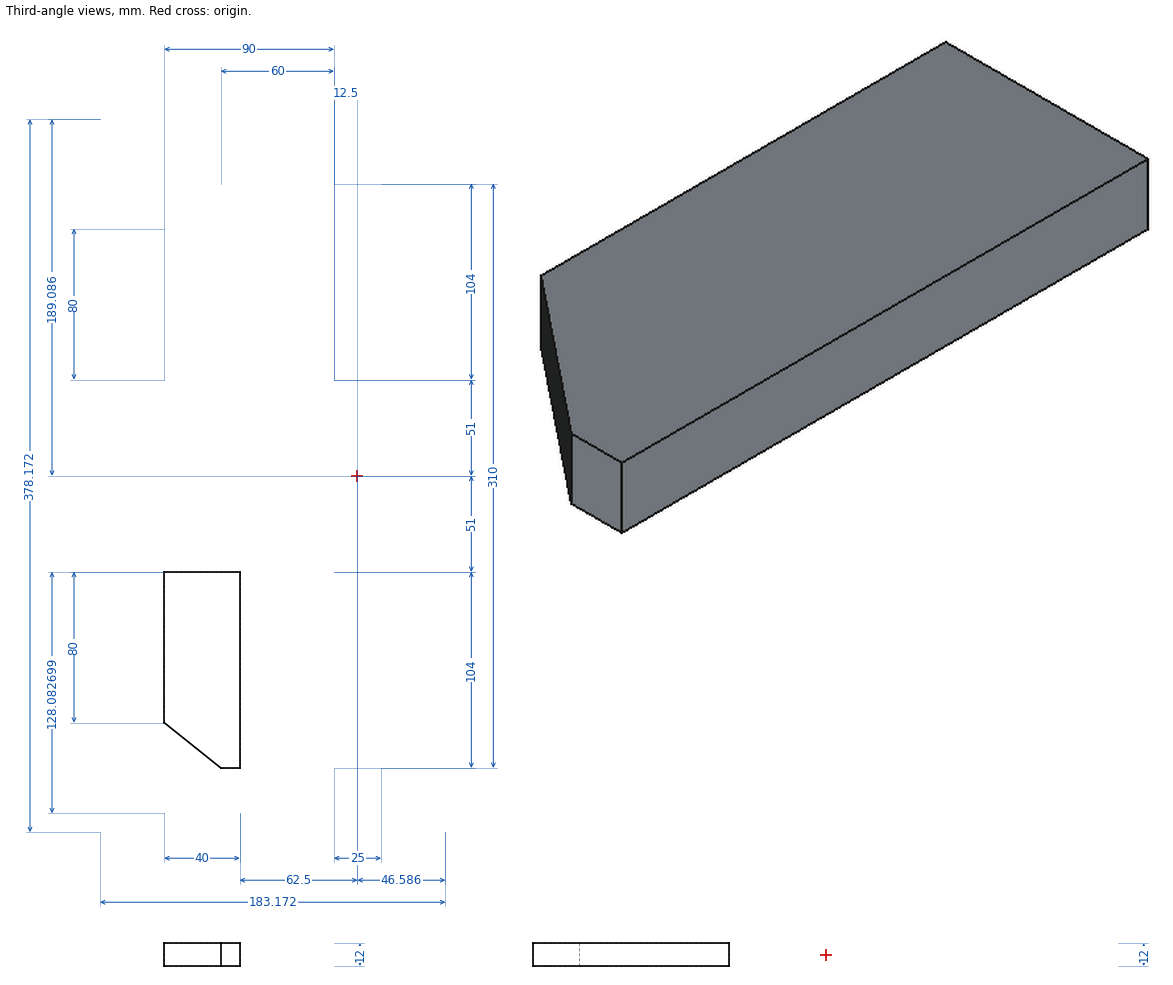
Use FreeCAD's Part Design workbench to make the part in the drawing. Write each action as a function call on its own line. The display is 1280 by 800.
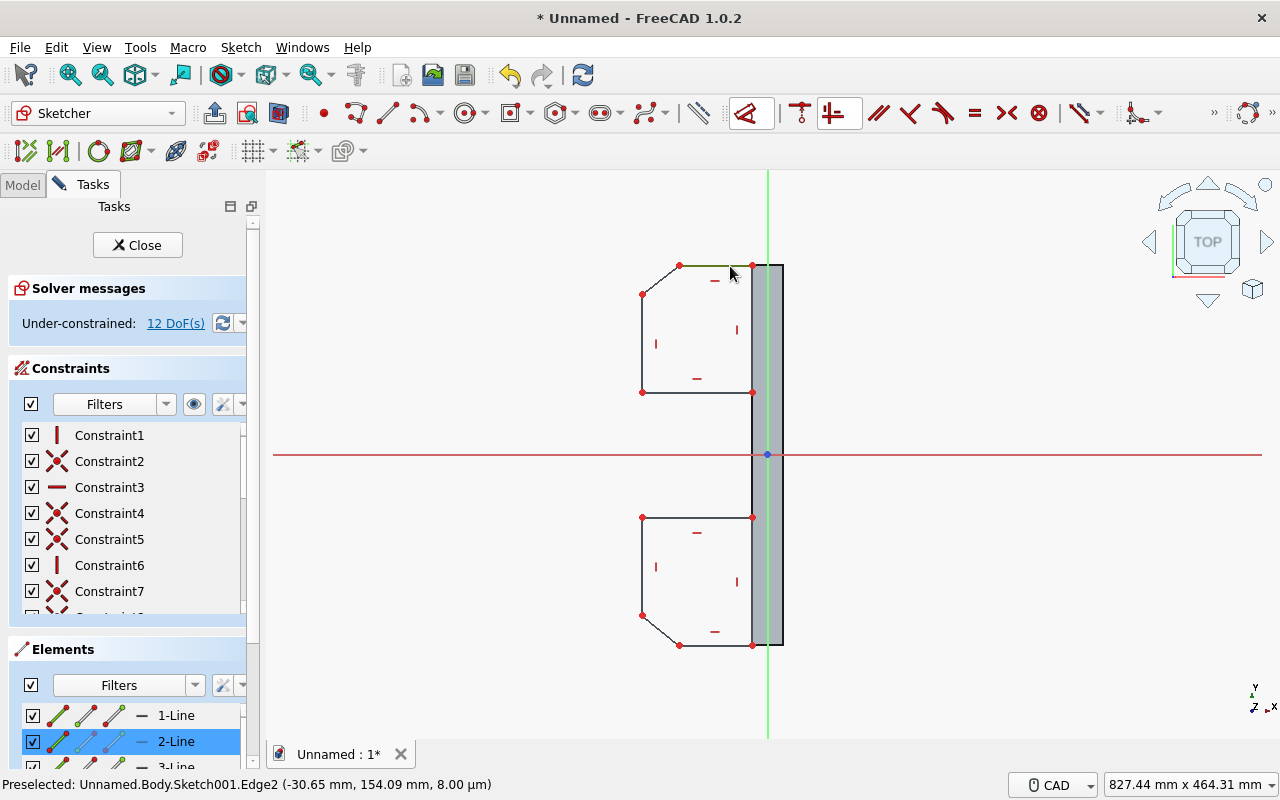
key(l)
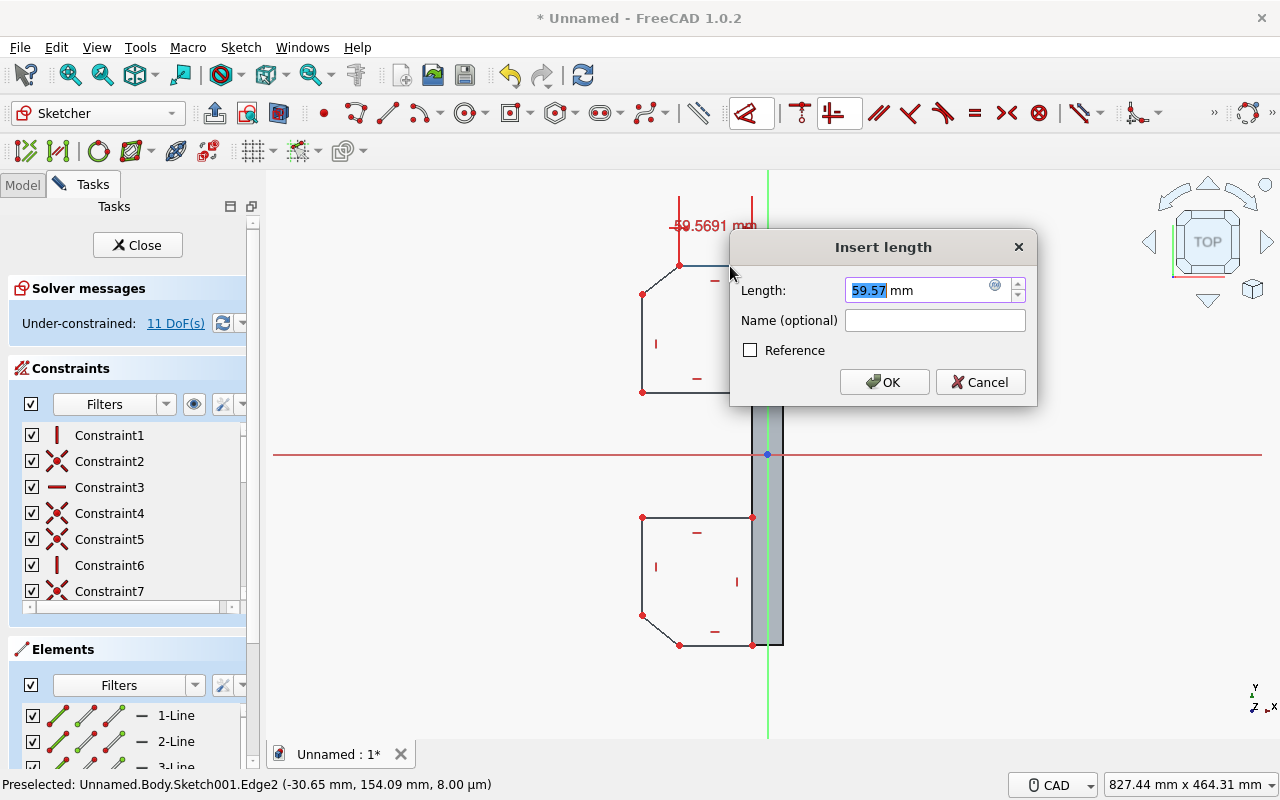
text(60)
key(Return)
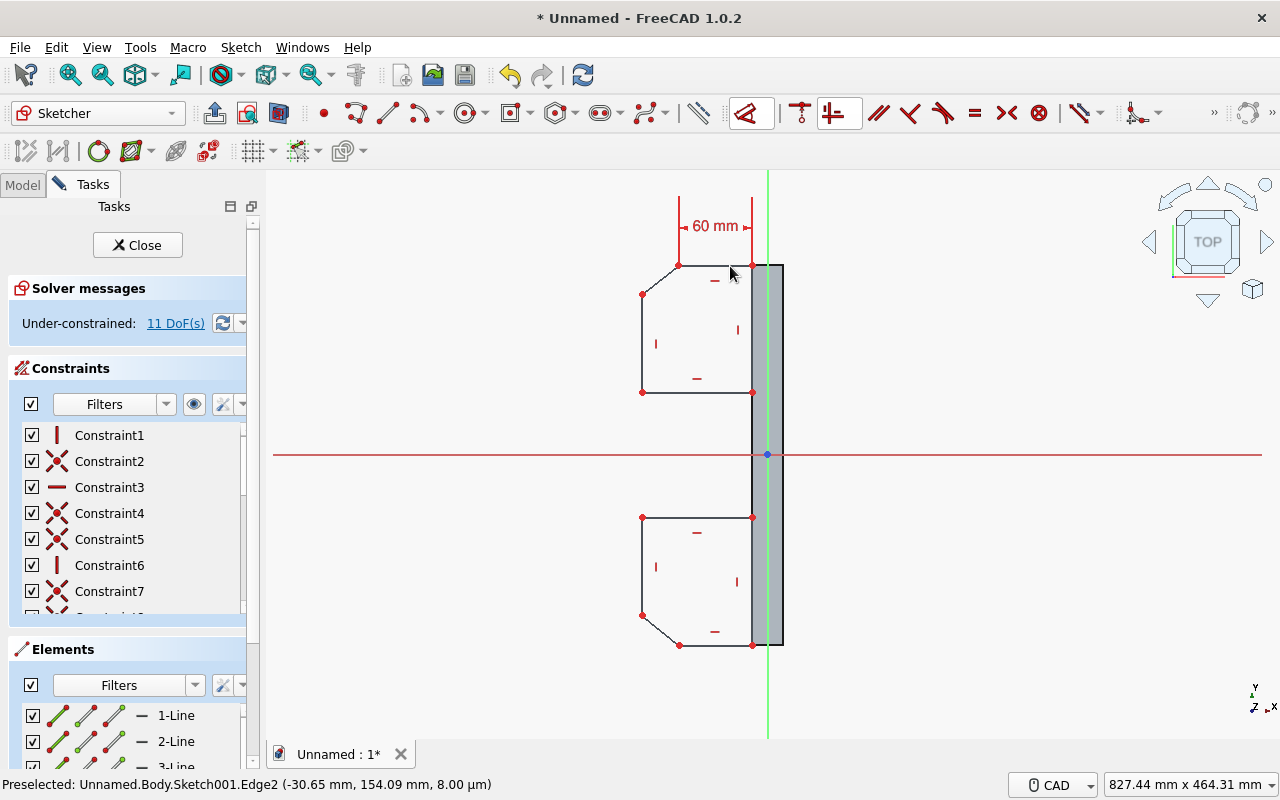
click(642, 324)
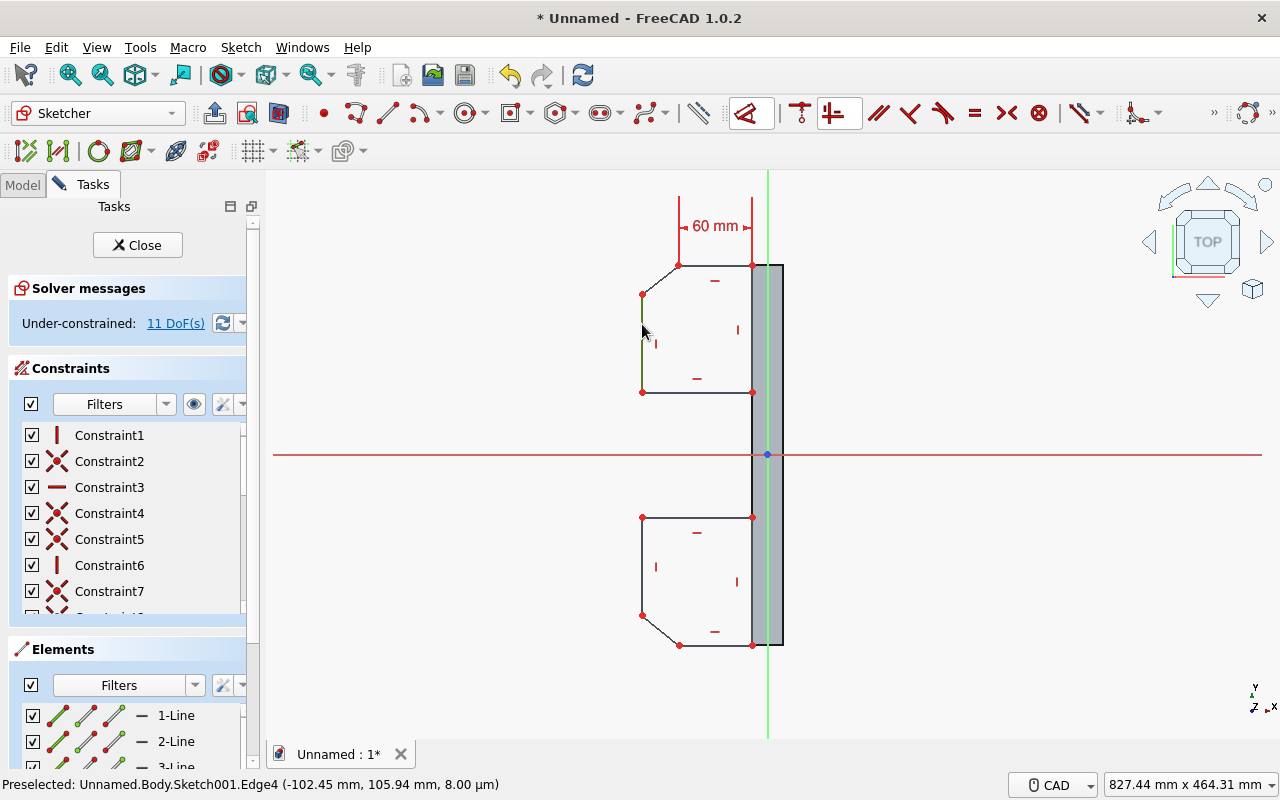
click(768, 114)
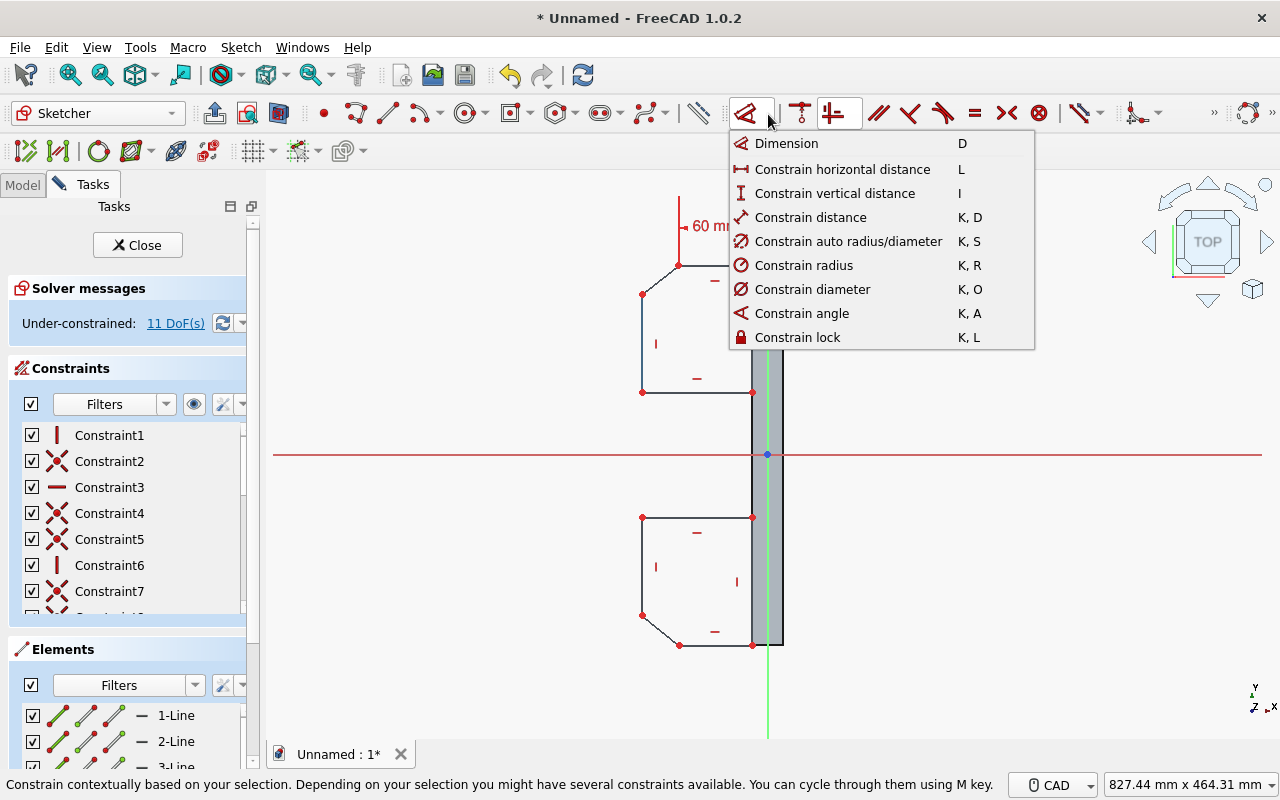
click(882, 193)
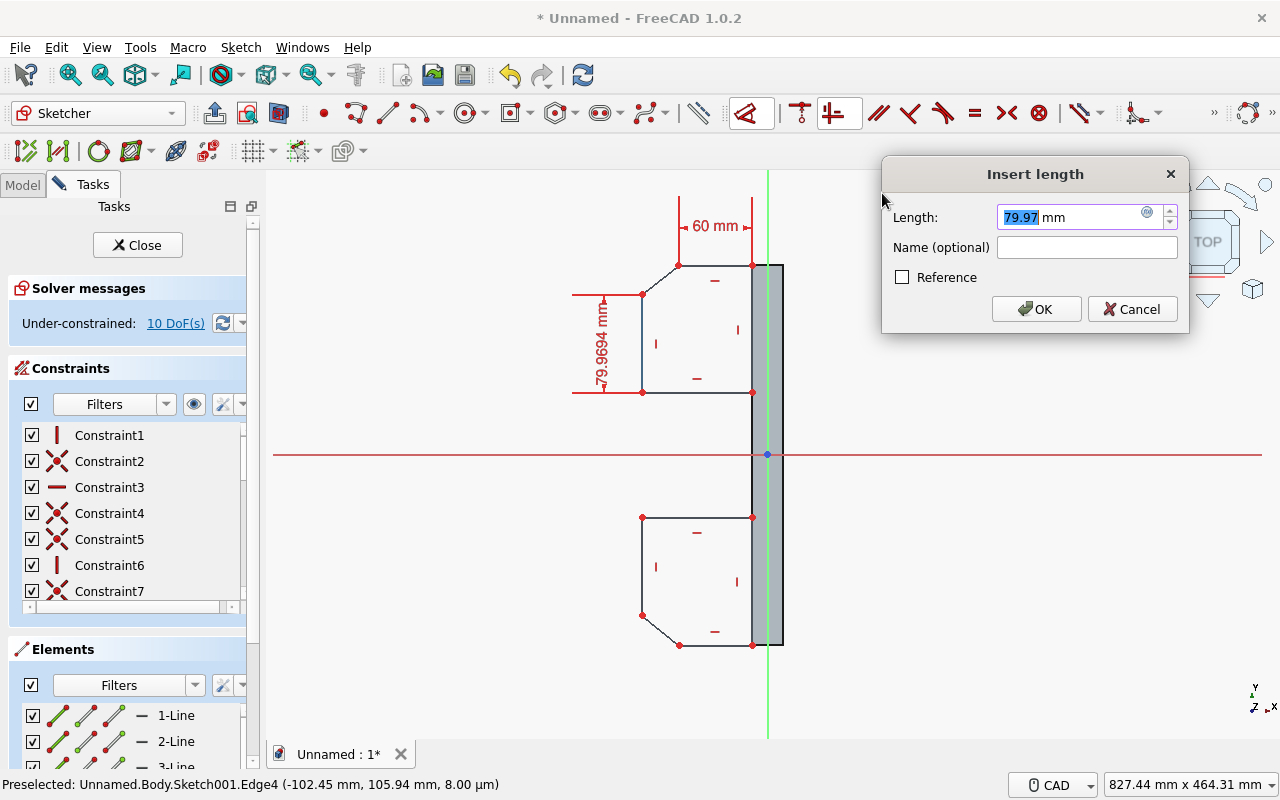
text(80)
key(Return)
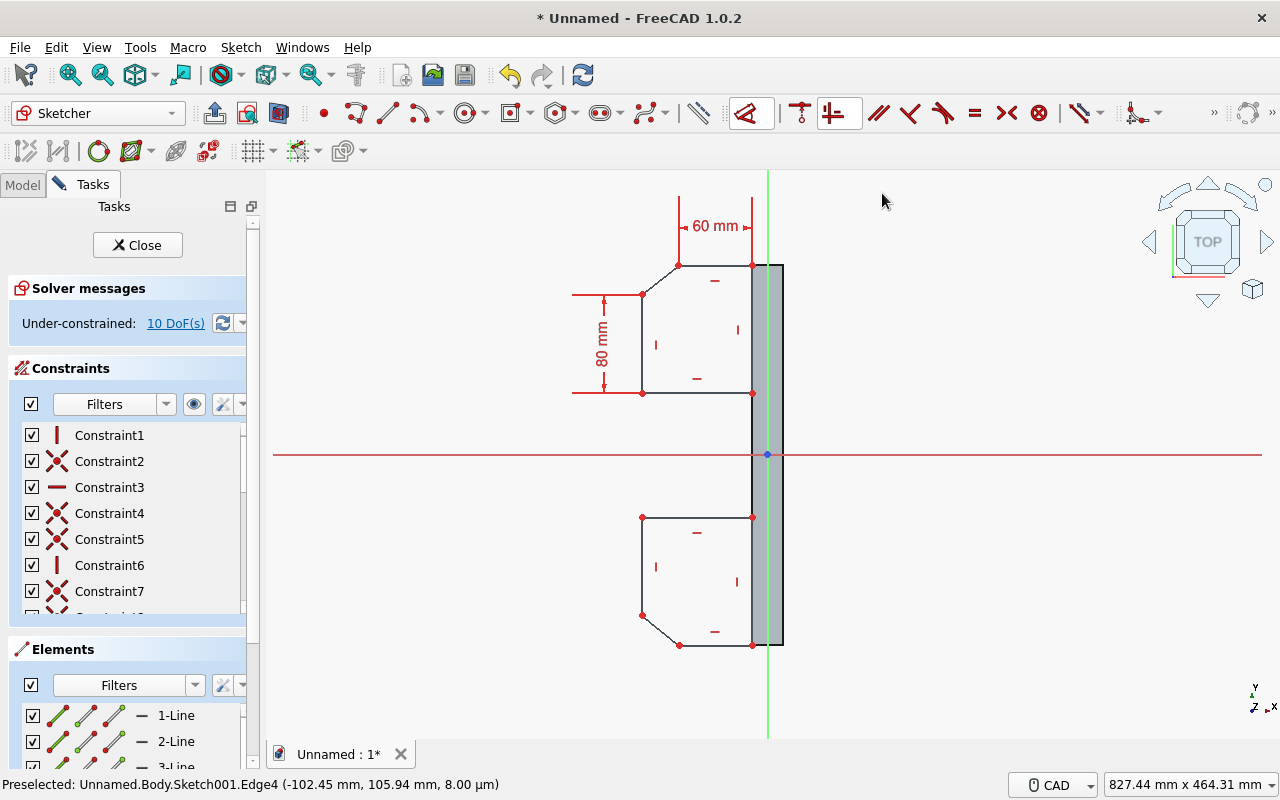
click(675, 393)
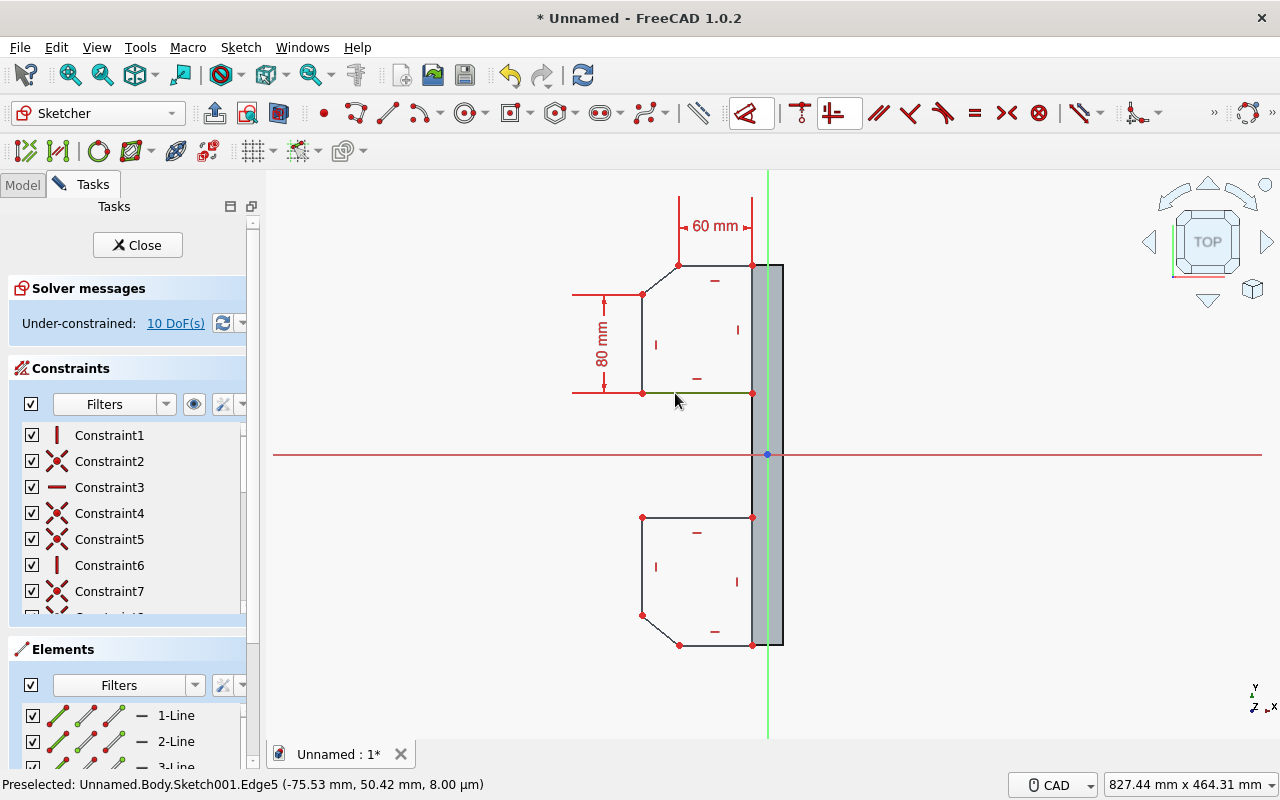
click(768, 114)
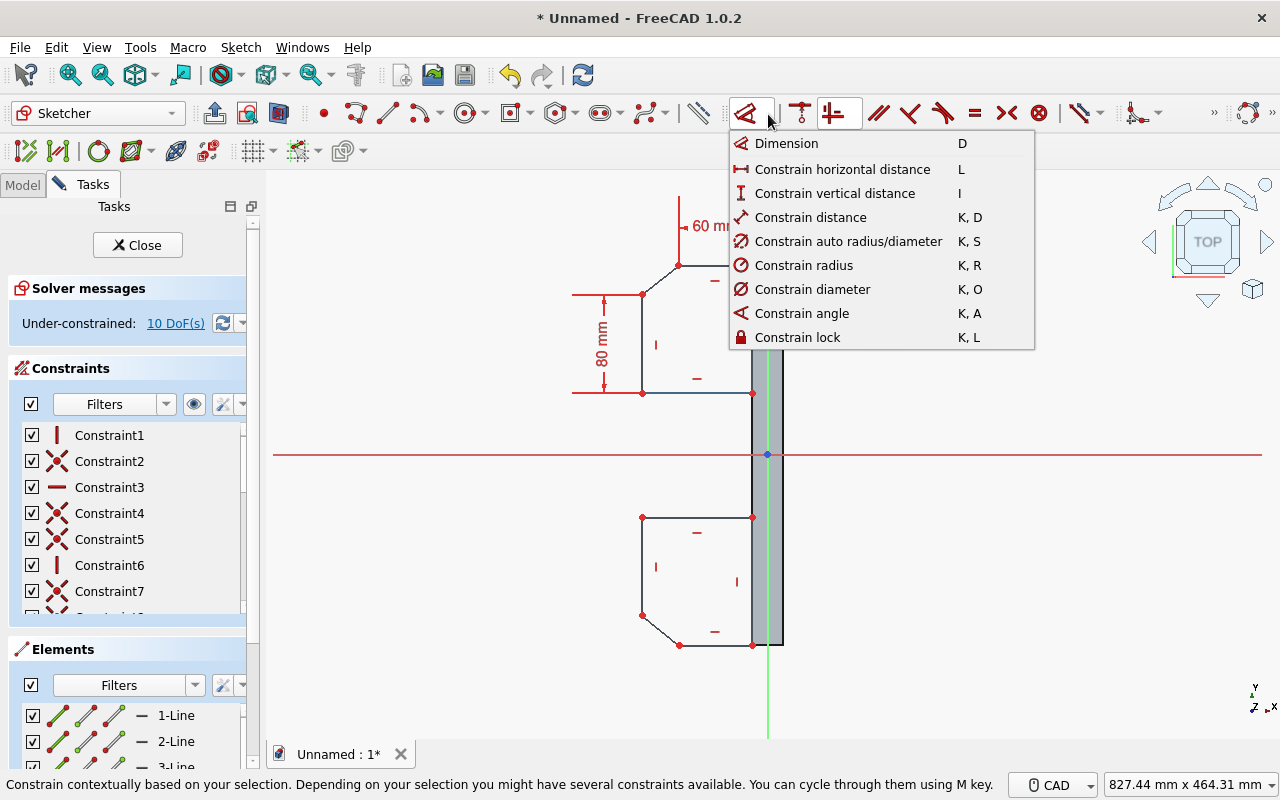
click(882, 169)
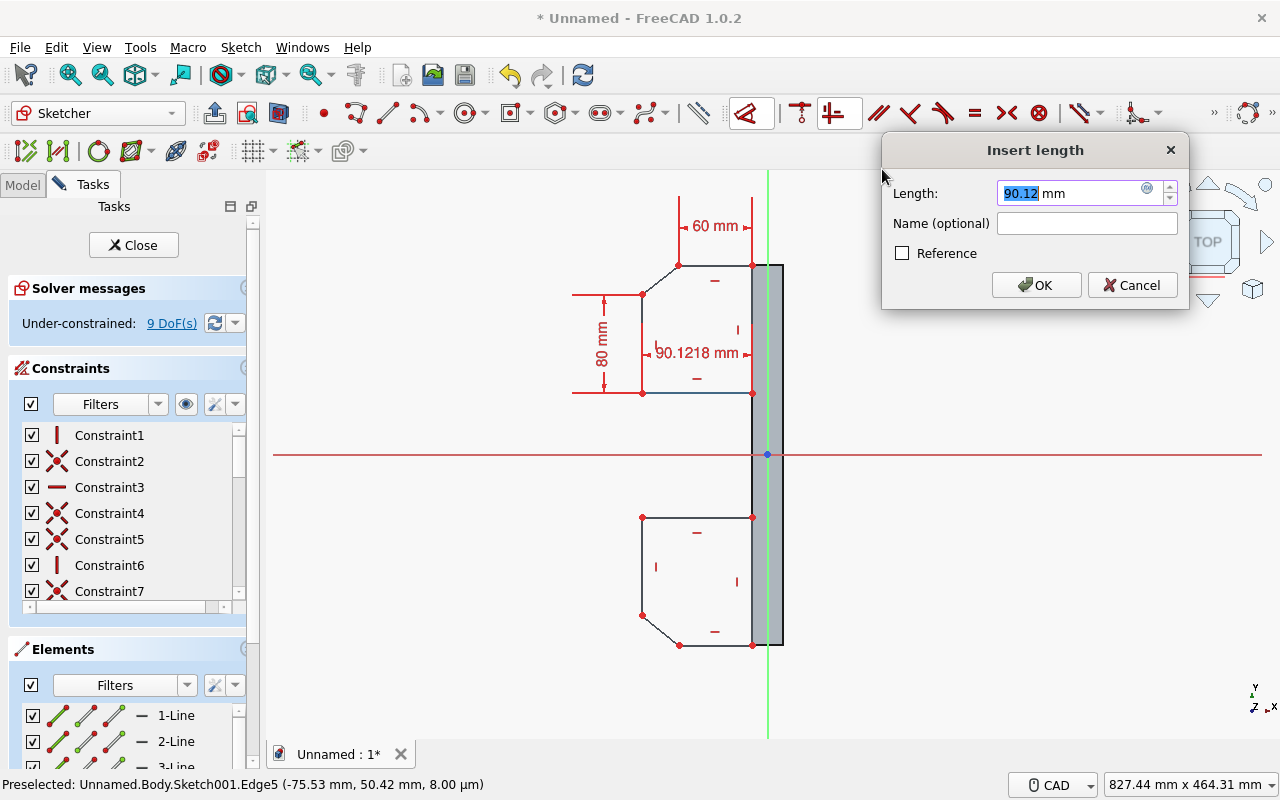
text(90)
key(Return)